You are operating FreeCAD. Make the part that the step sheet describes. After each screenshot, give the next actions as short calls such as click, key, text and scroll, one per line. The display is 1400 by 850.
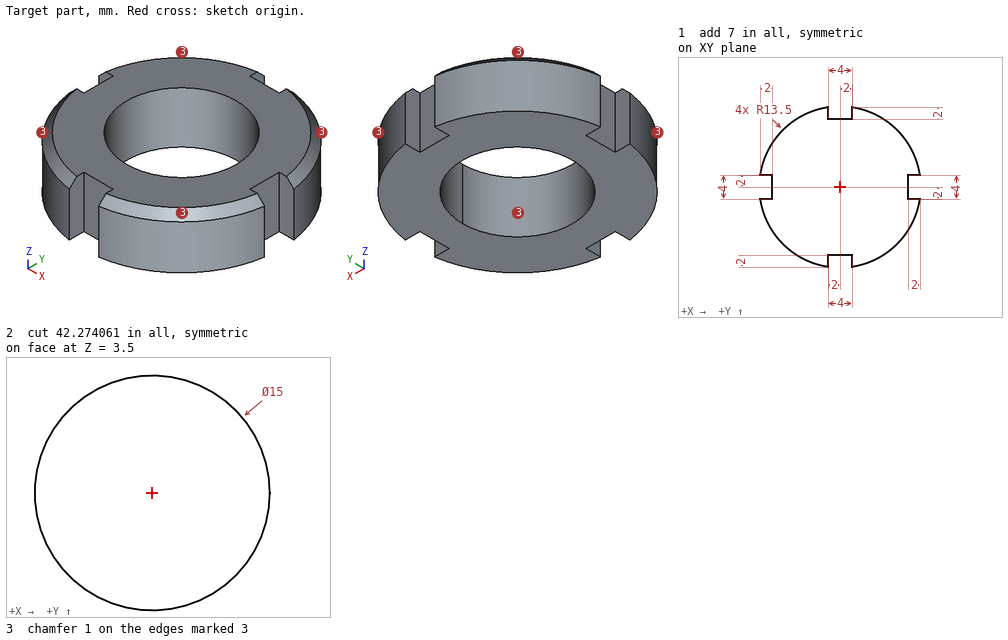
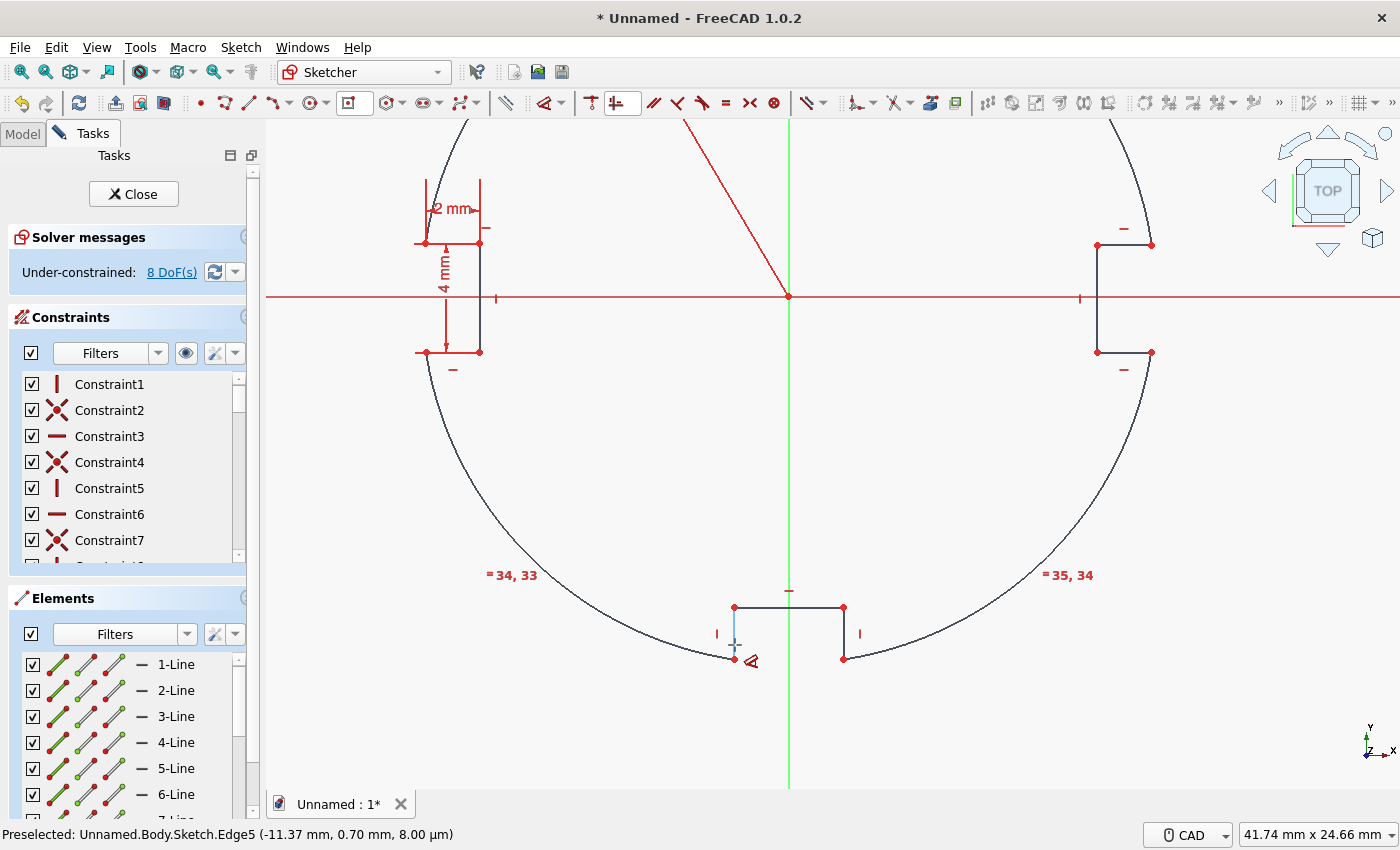
click(734, 644)
click(700, 634)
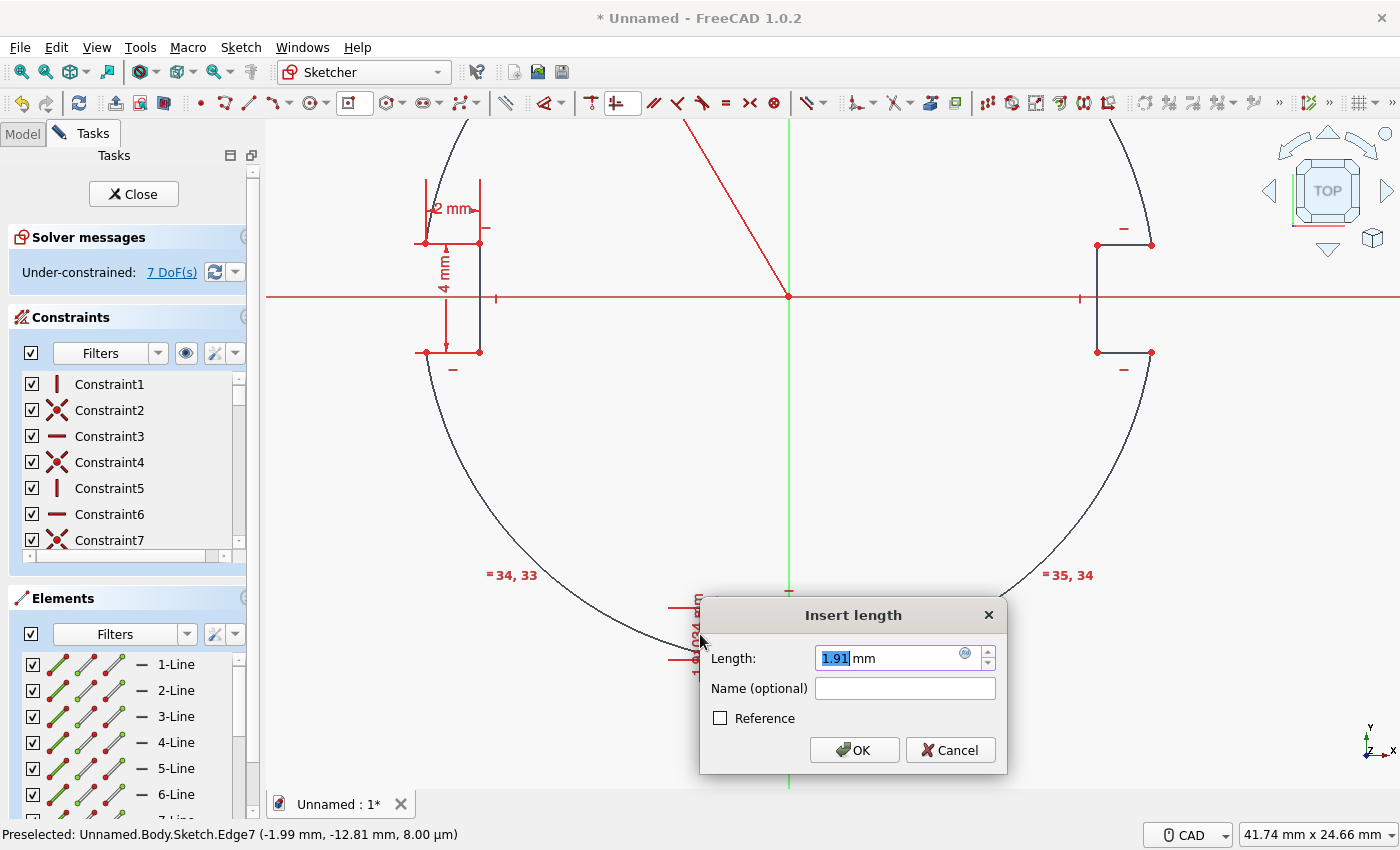
text(2)
key(Return)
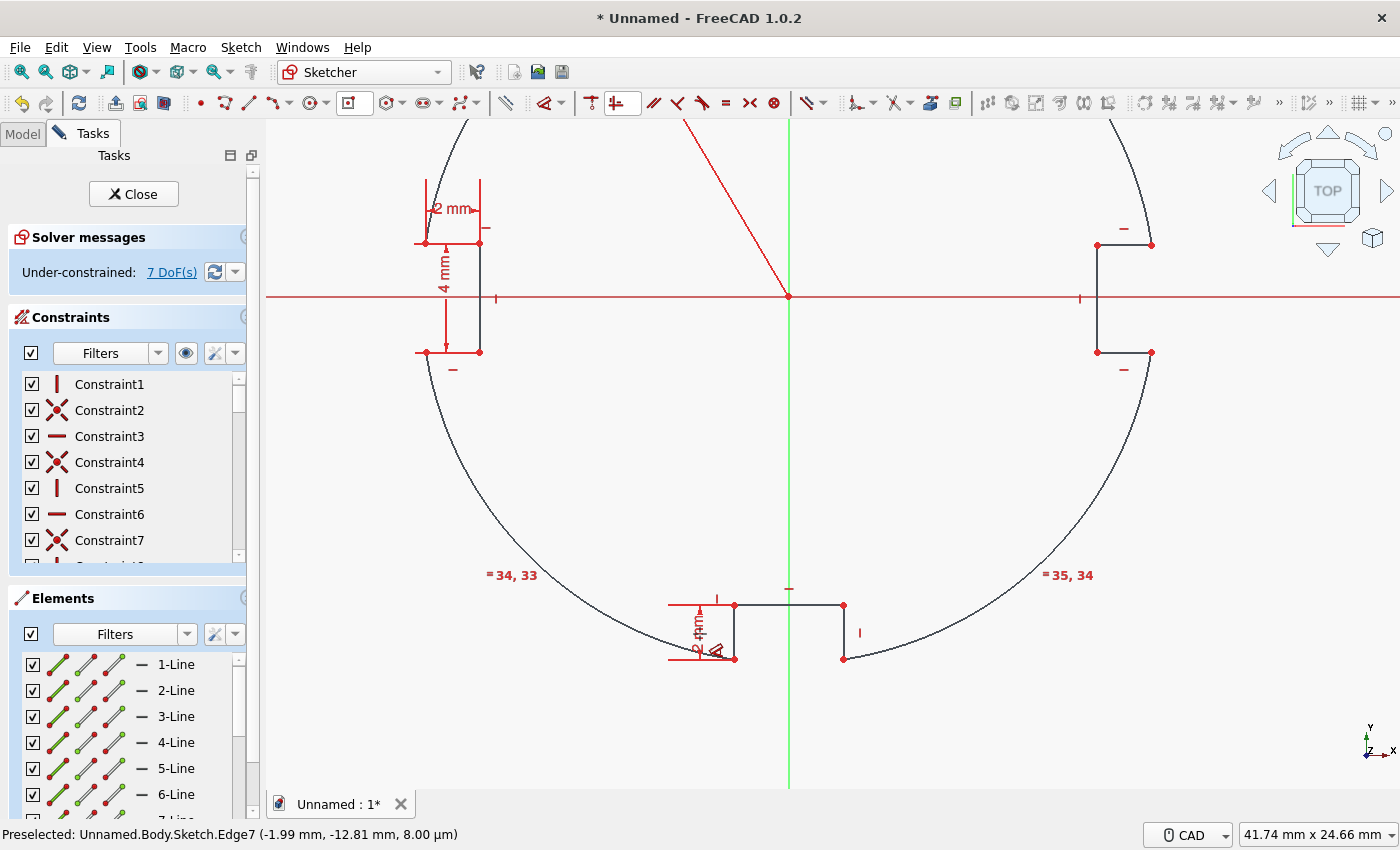
click(767, 605)
click(814, 639)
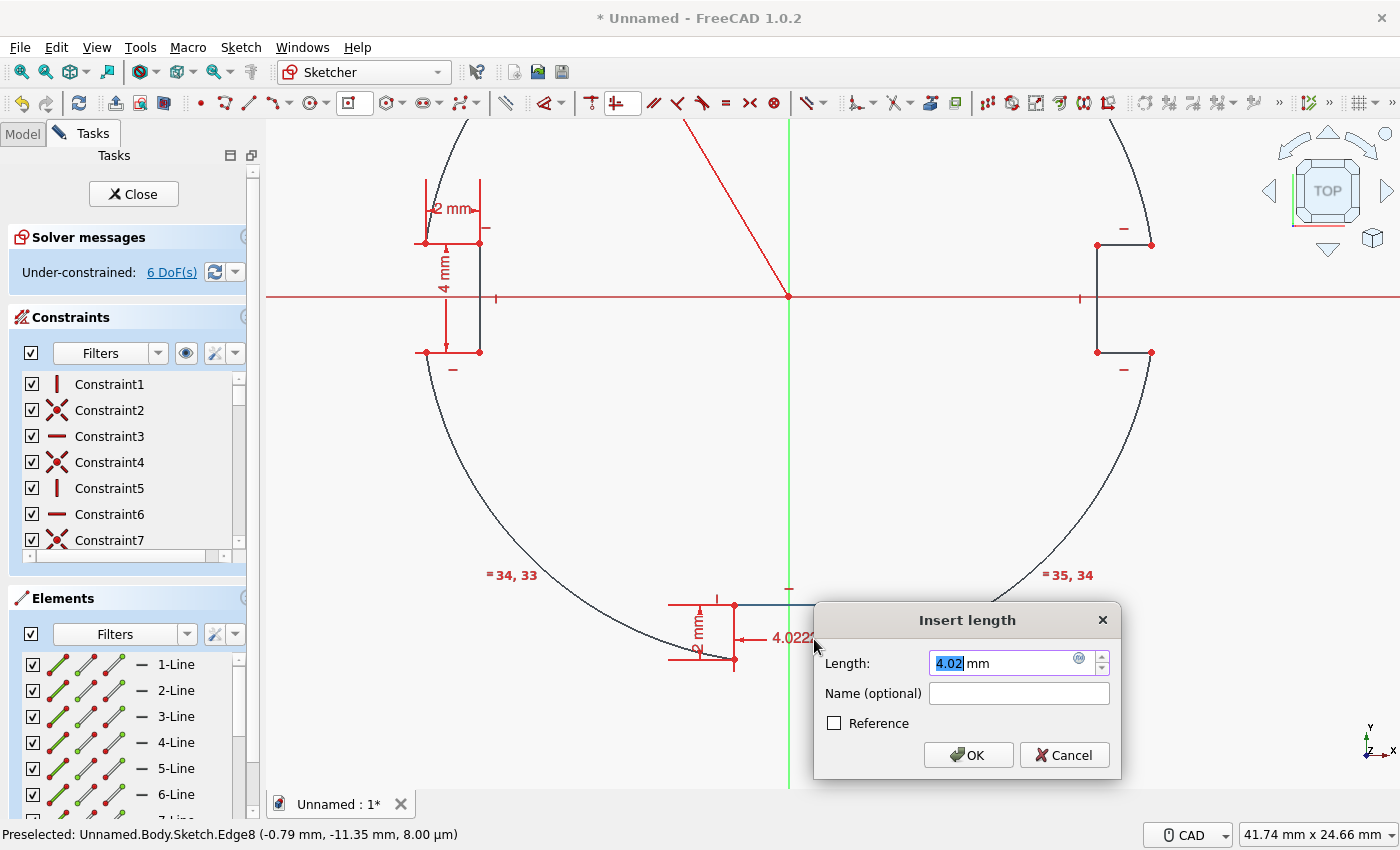
text(4)
key(Return)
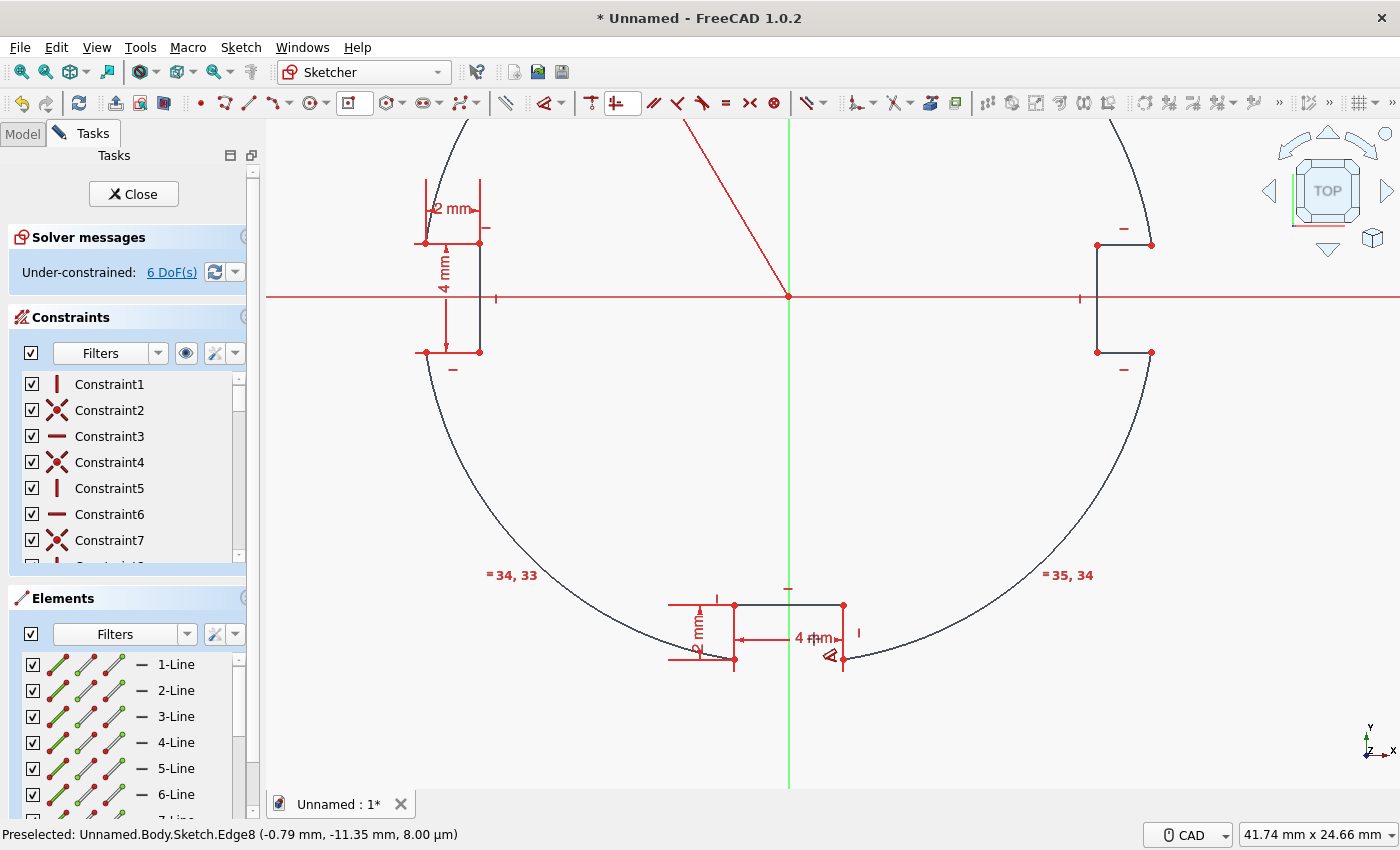
click(1135, 353)
click(1124, 387)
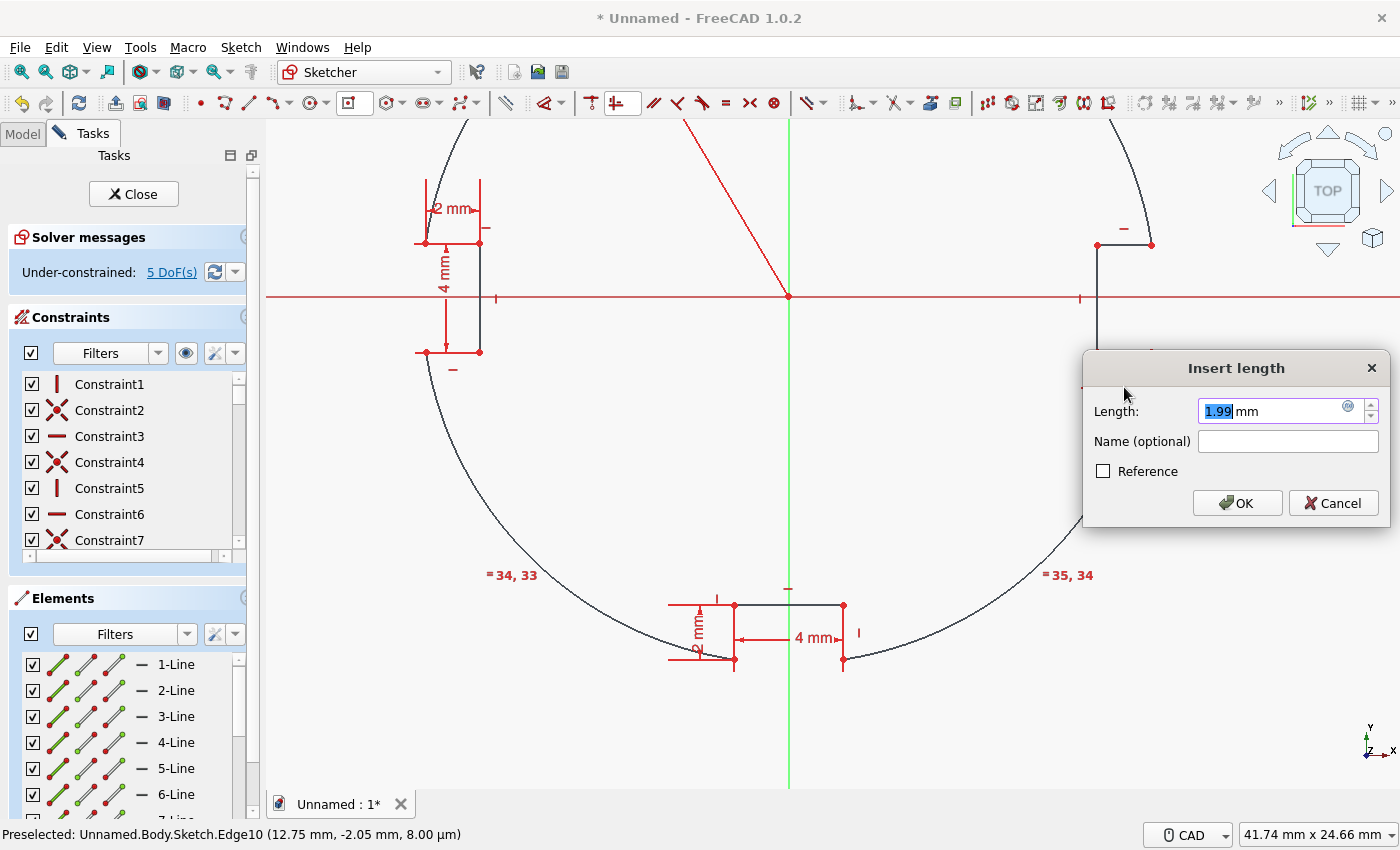
text(2)
key(Return)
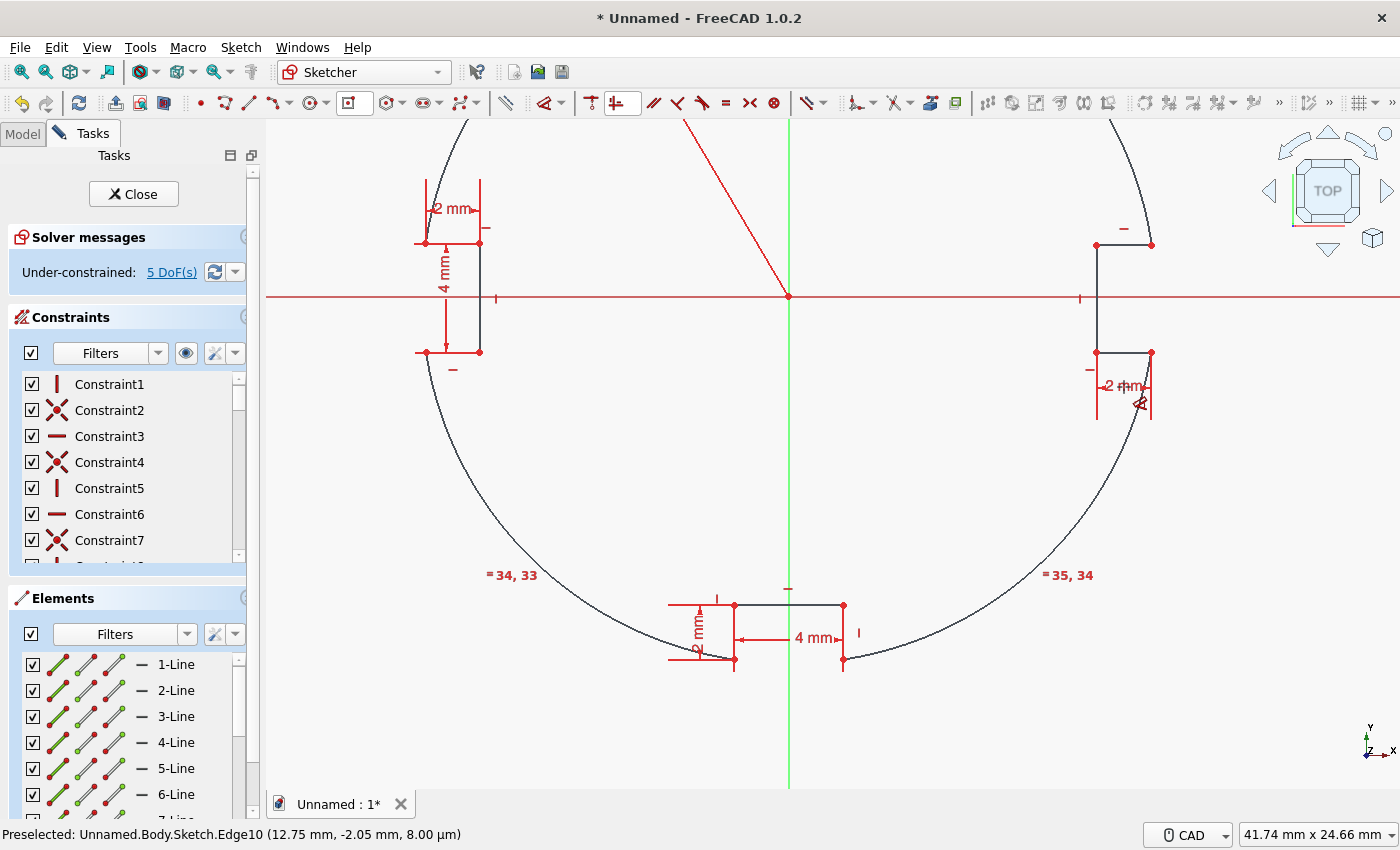
click(1097, 320)
click(1131, 274)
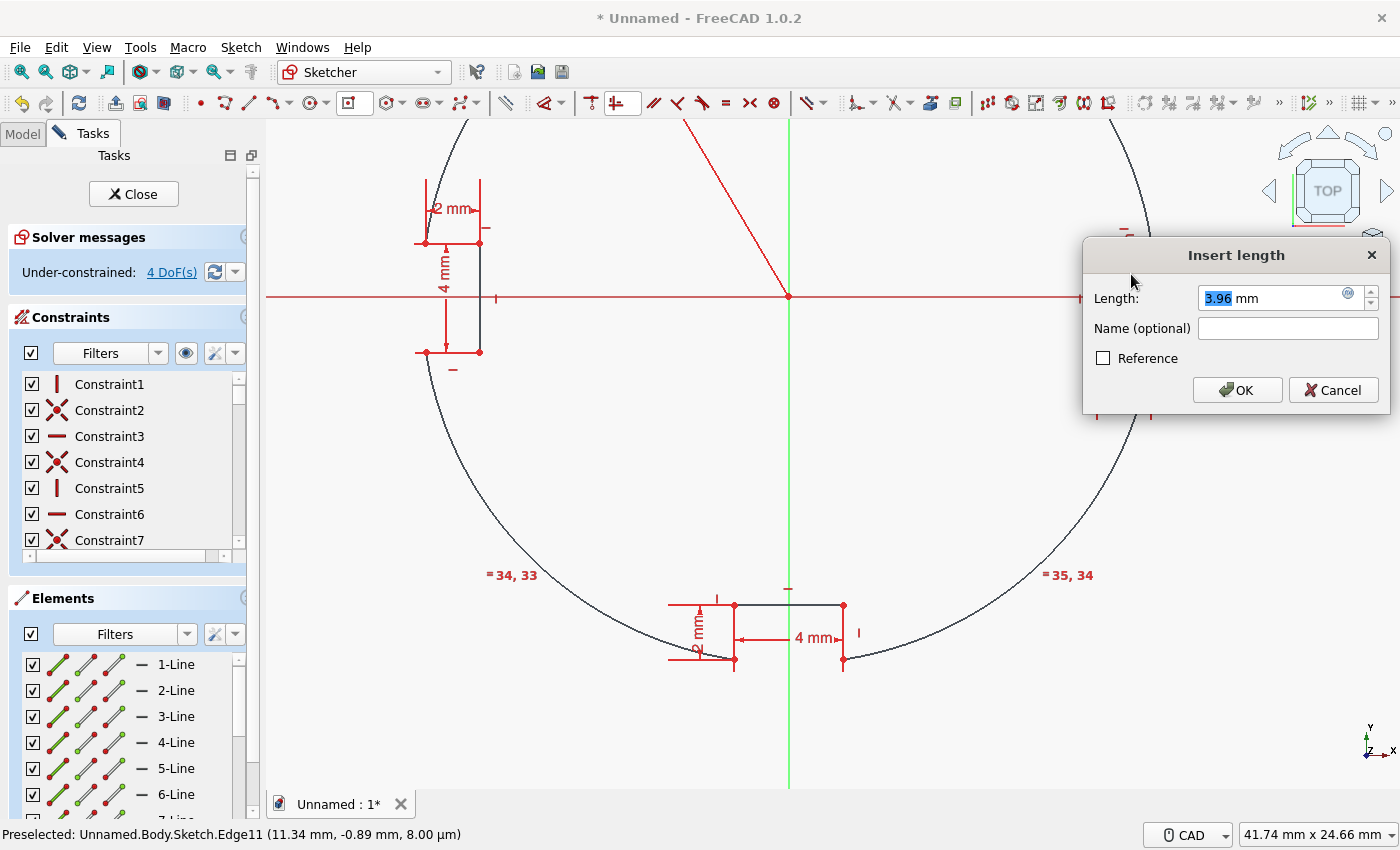
text(4)
key(Return)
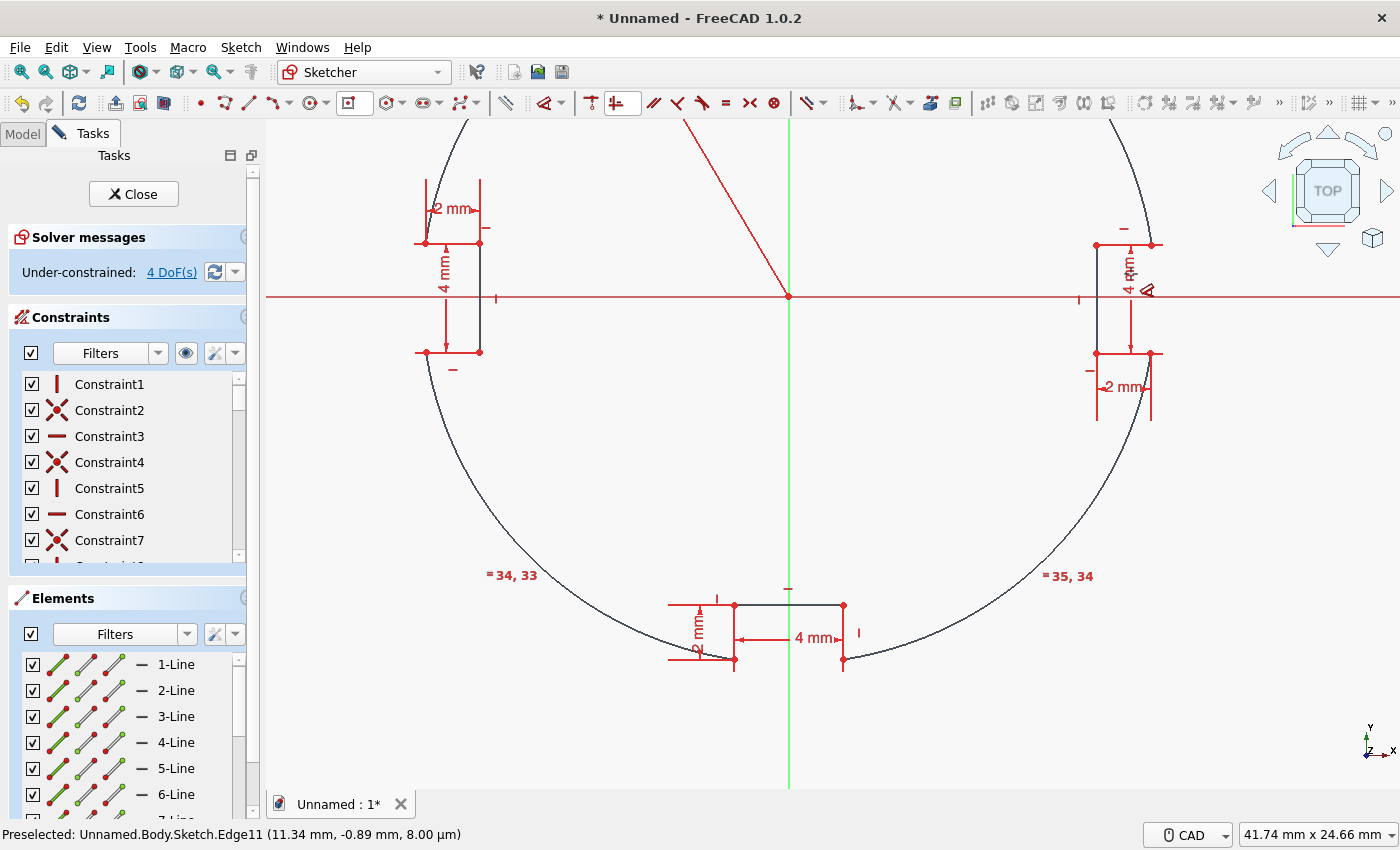
scroll(735, 645, down, 3)